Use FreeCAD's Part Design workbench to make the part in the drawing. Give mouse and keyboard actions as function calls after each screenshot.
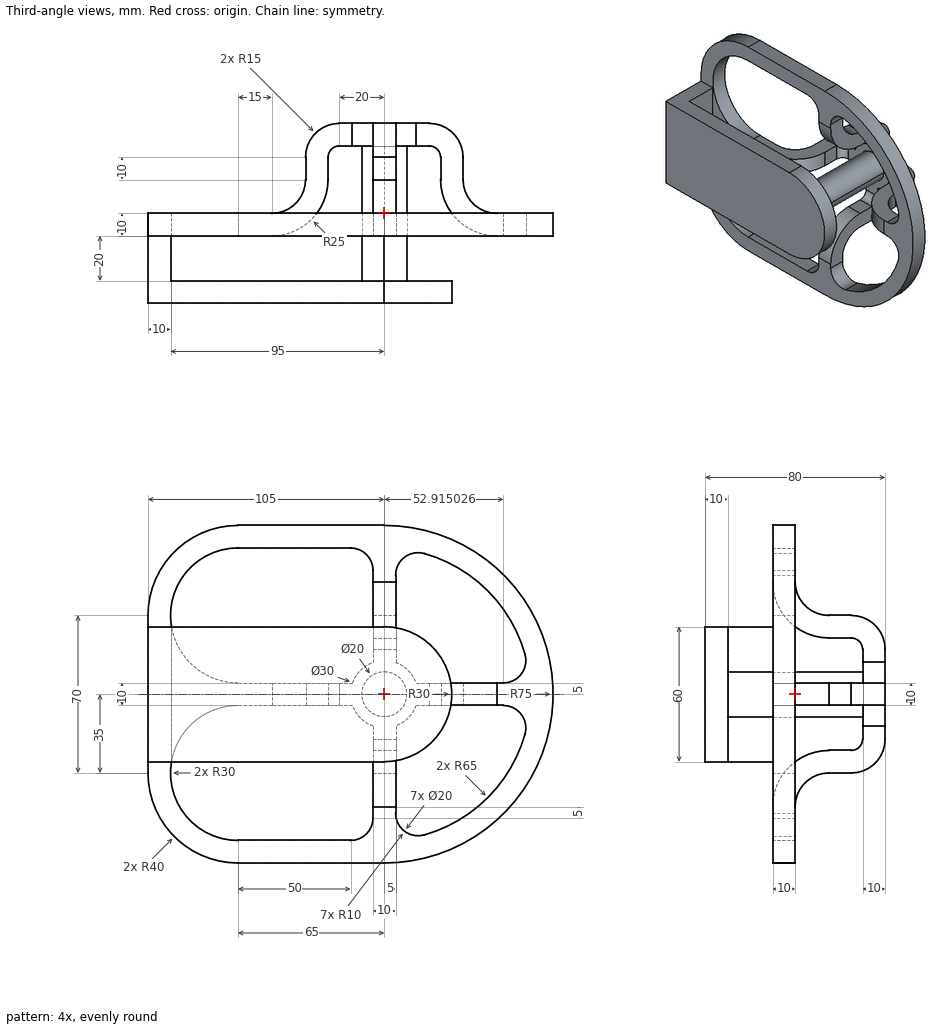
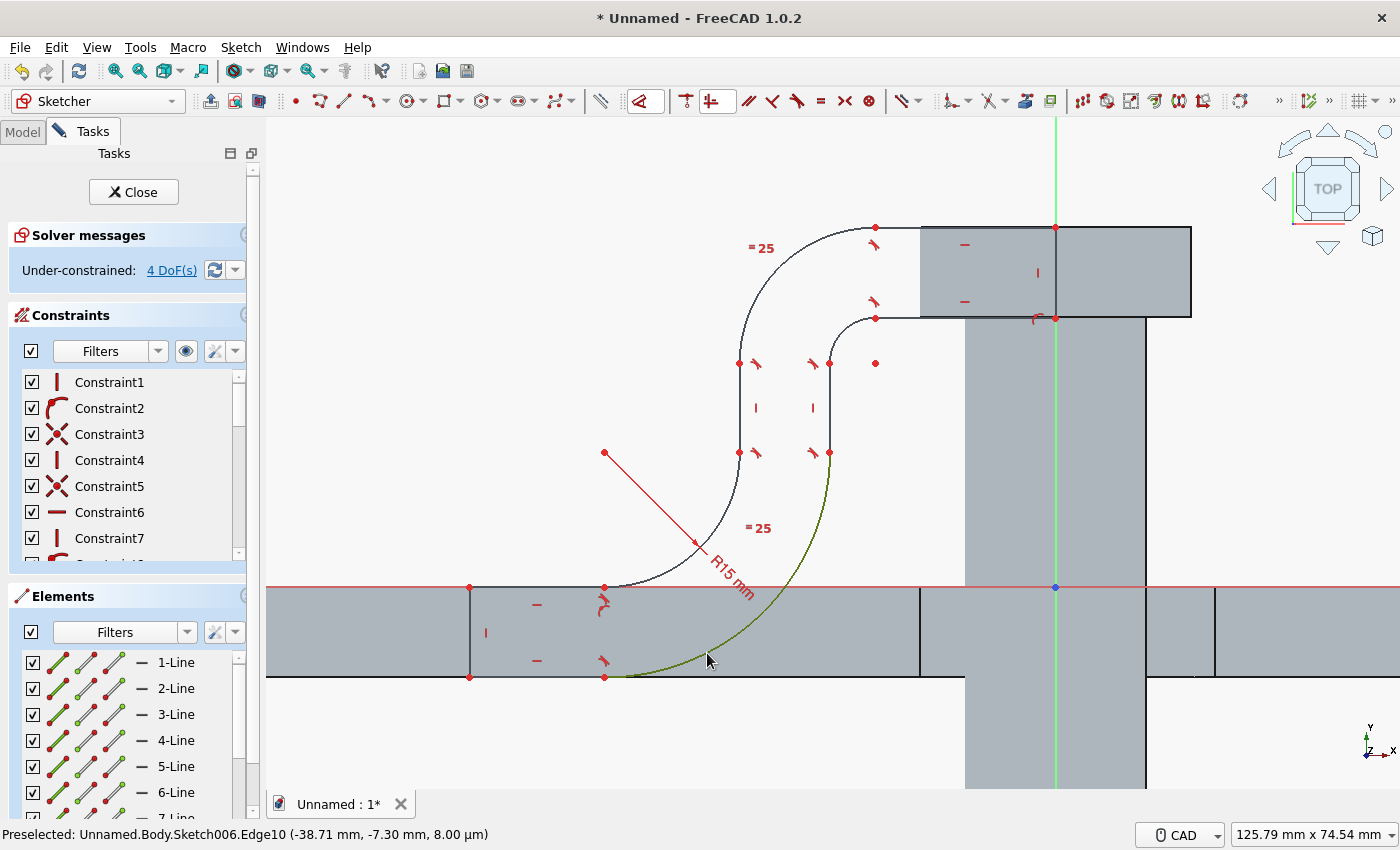
click(658, 102)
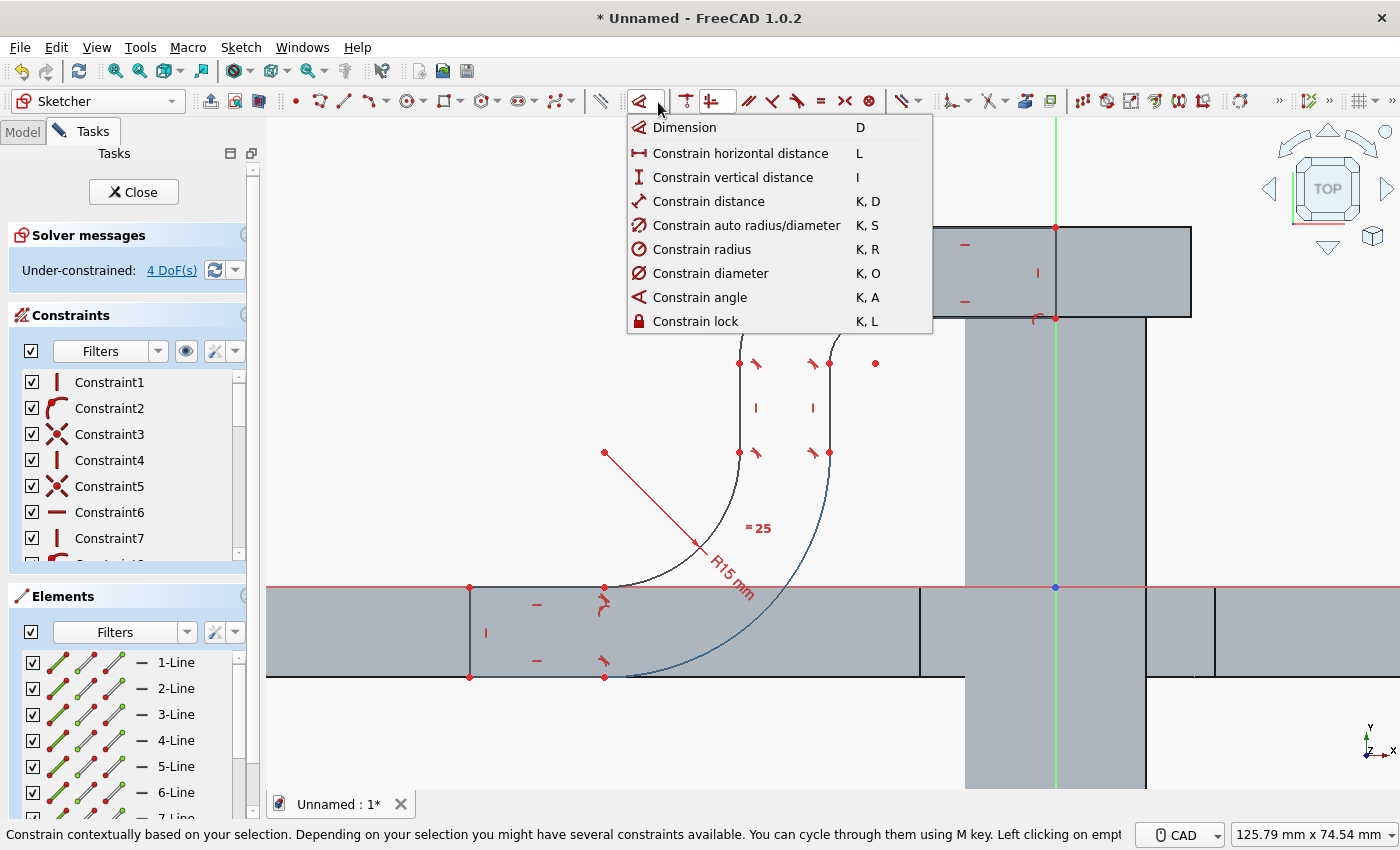
click(780, 249)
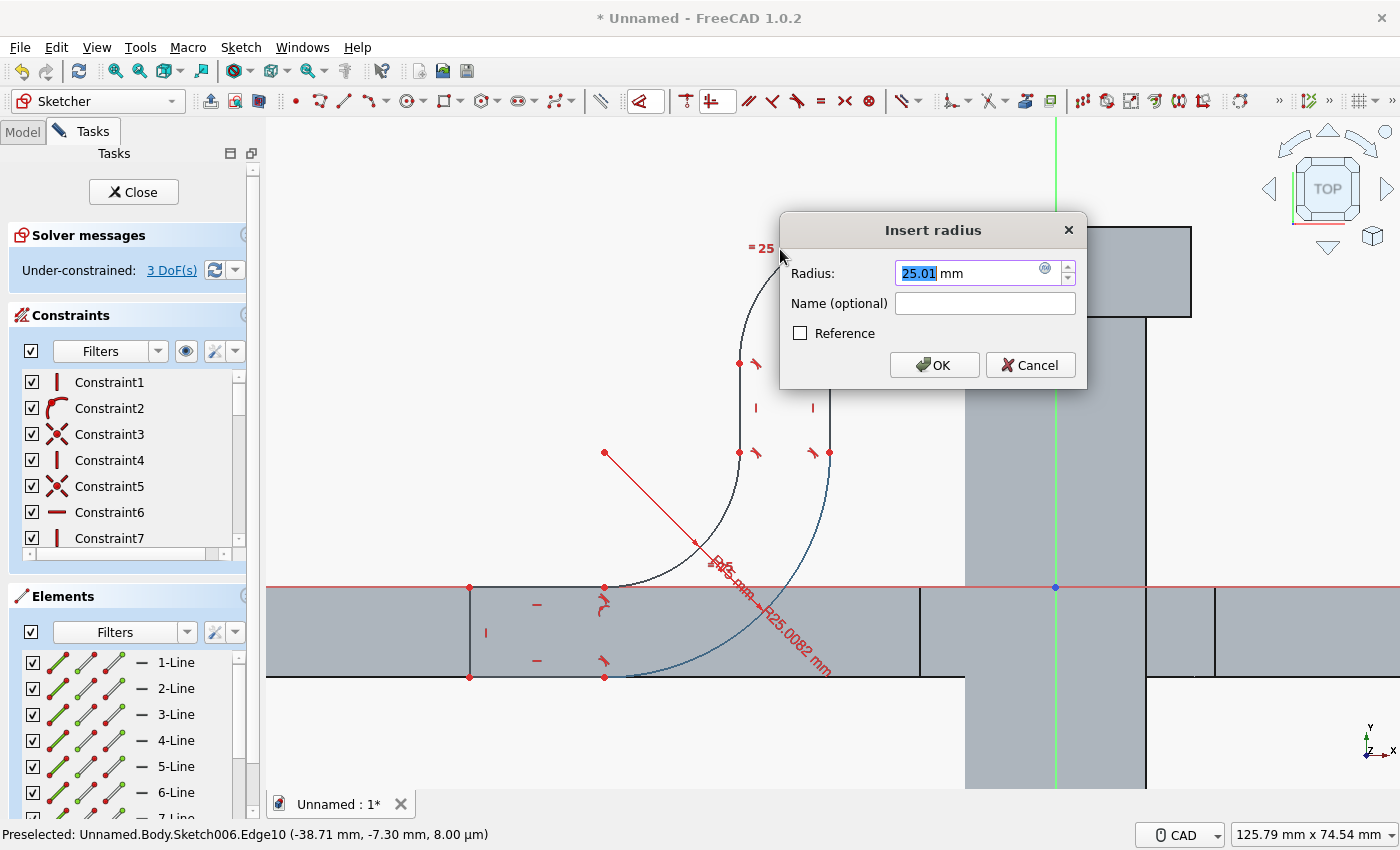
text(25)
key(Return)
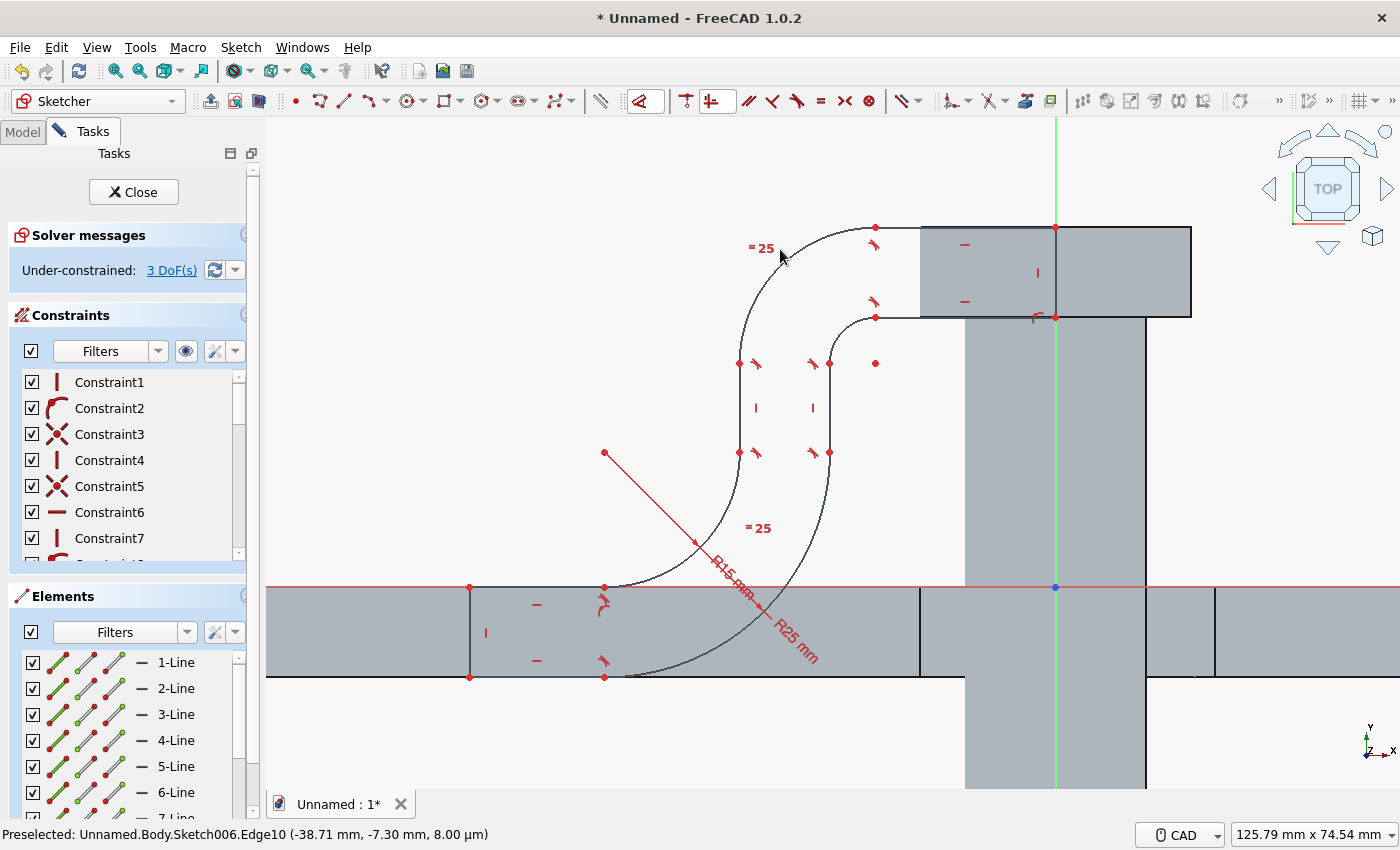
click(740, 390)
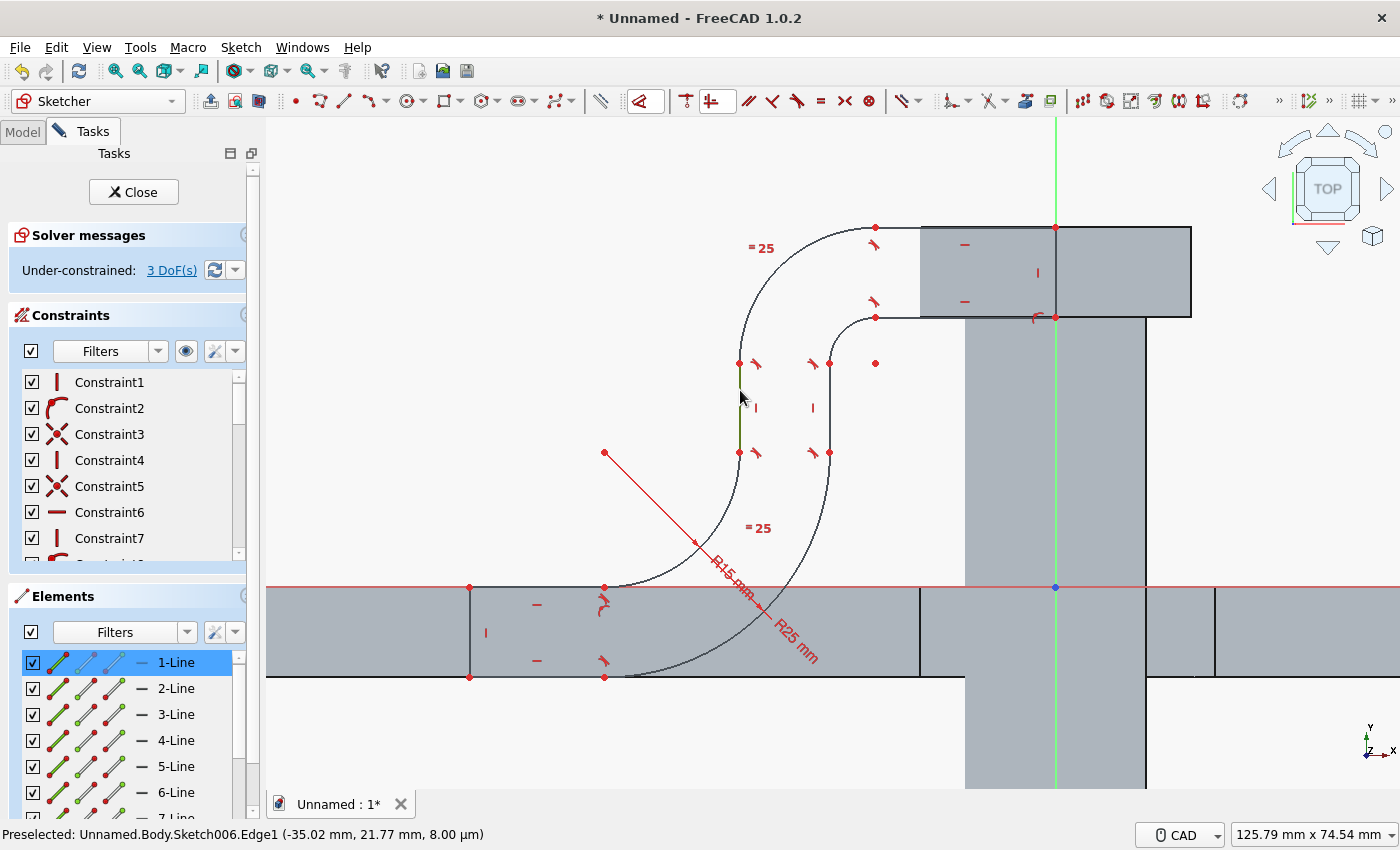
key(i)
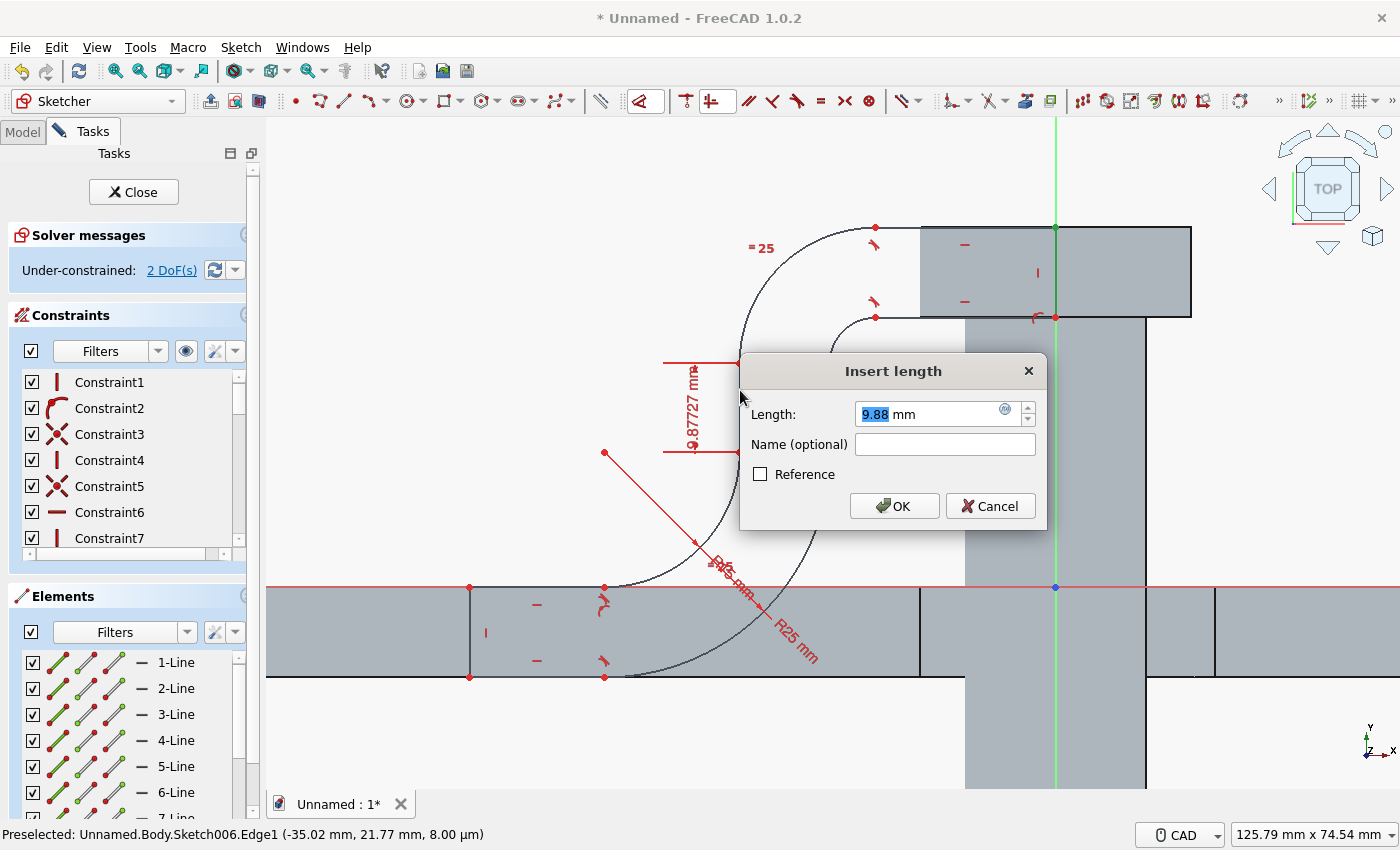
text(10)
key(Return)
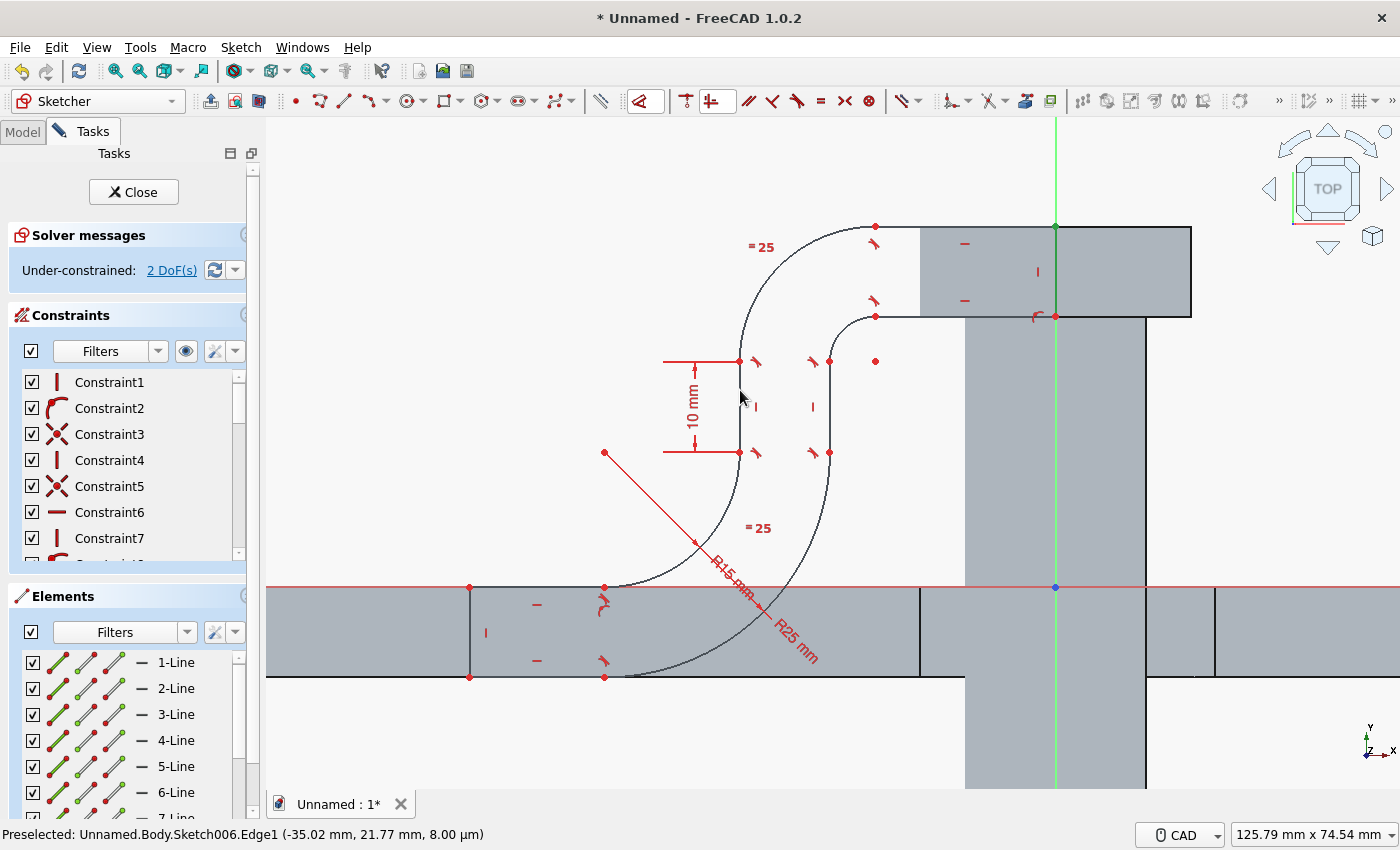
click(564, 587)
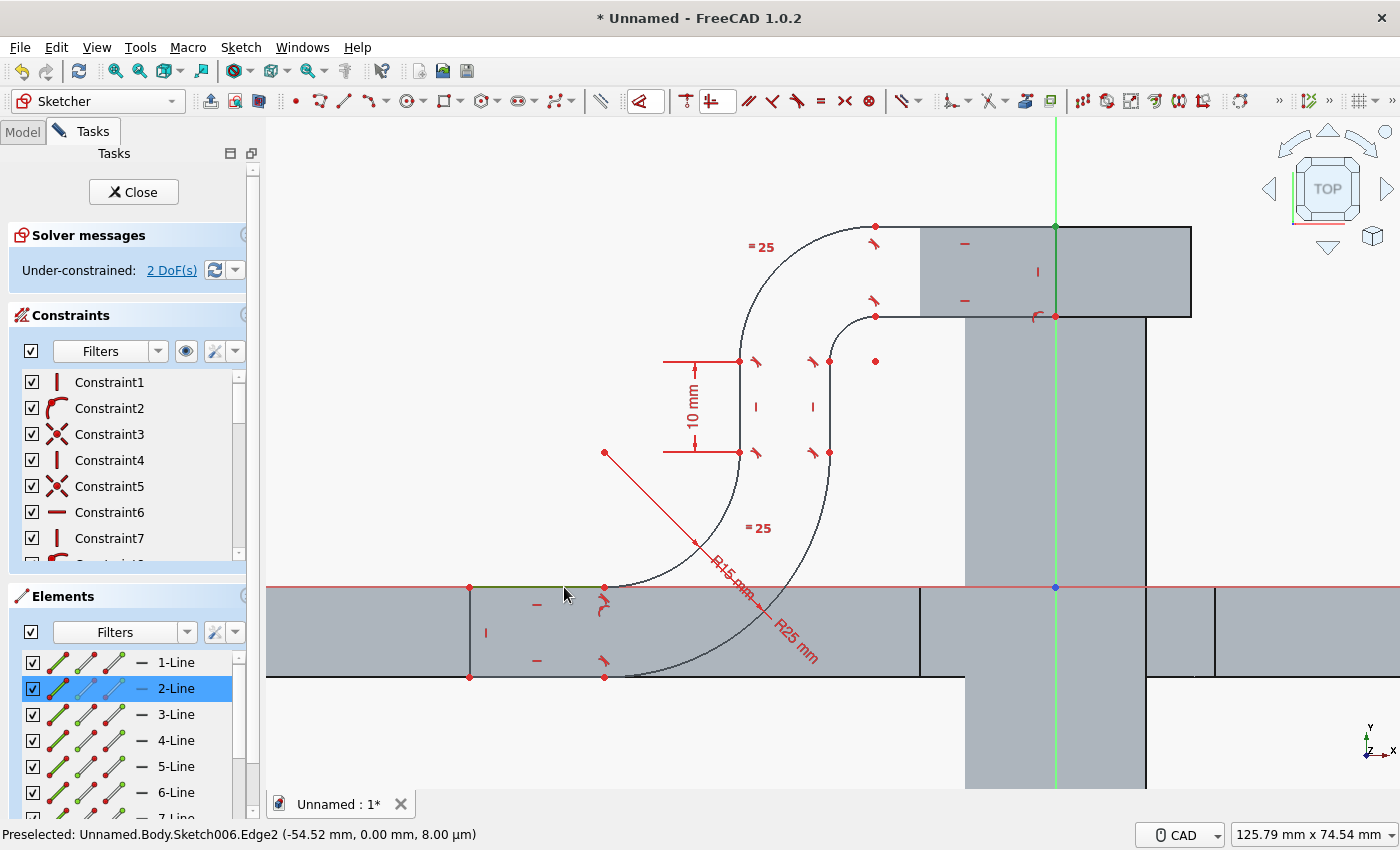
click(658, 102)